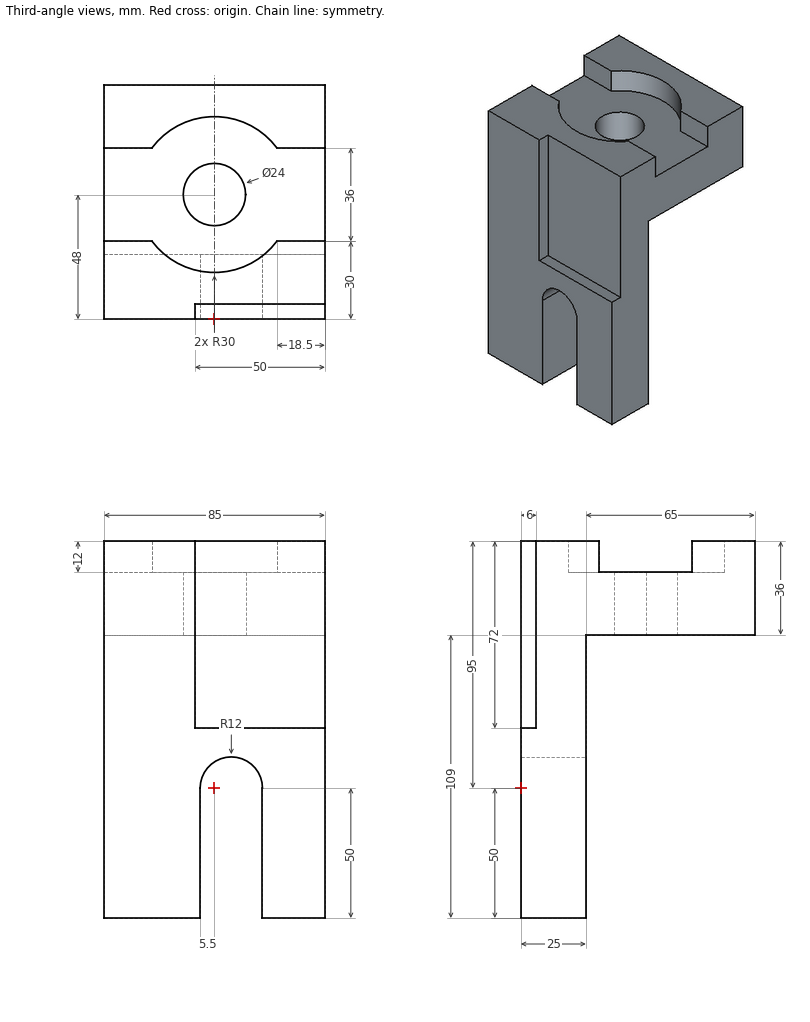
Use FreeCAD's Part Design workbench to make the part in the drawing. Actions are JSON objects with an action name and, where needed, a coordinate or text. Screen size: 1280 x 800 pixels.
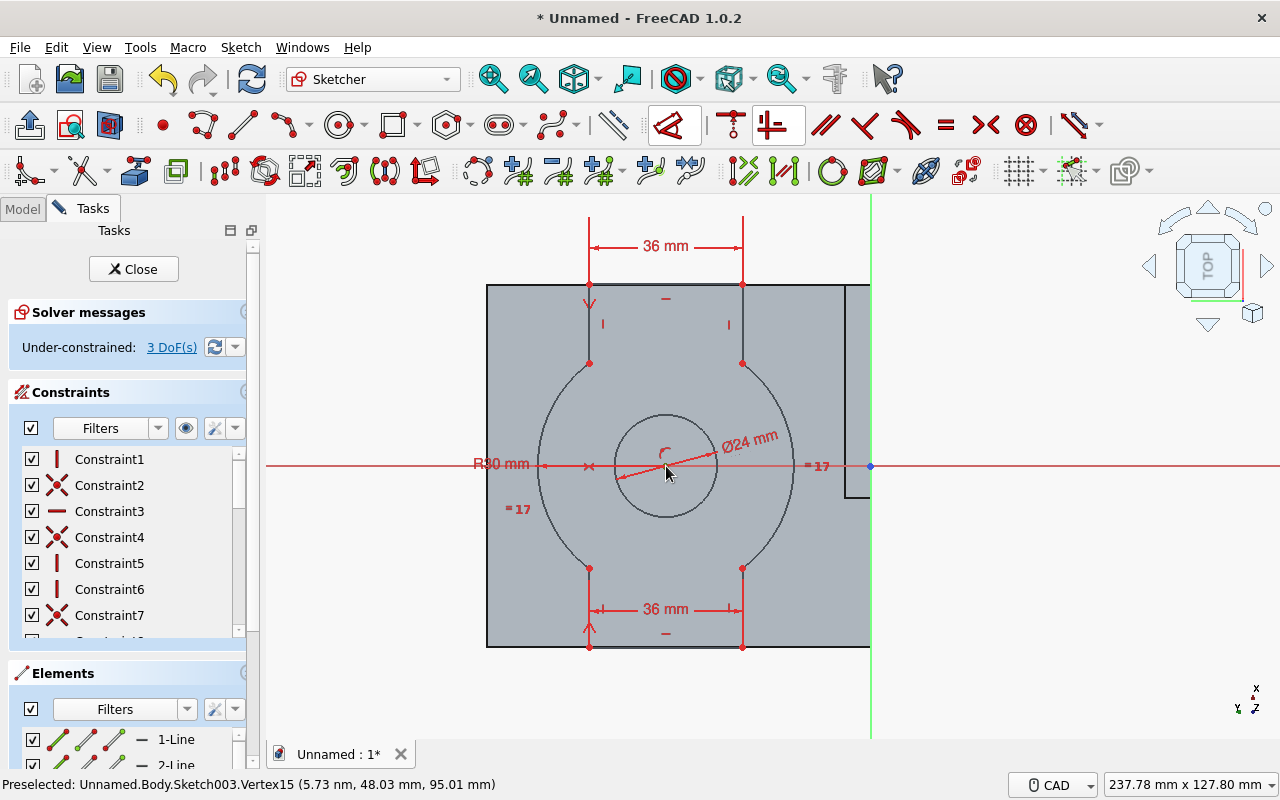
{"action": "left_click", "coordinate": [696, 126]}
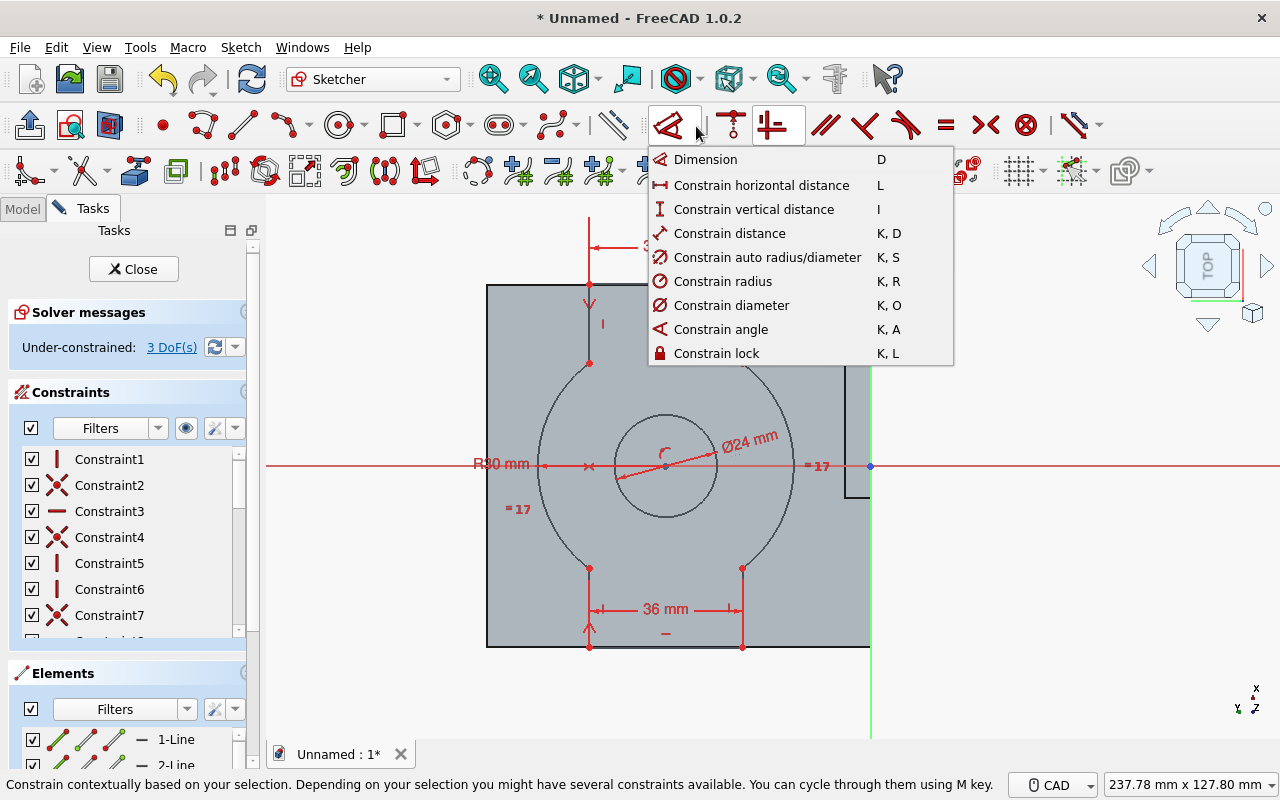
{"action": "left_click", "coordinate": [801, 185]}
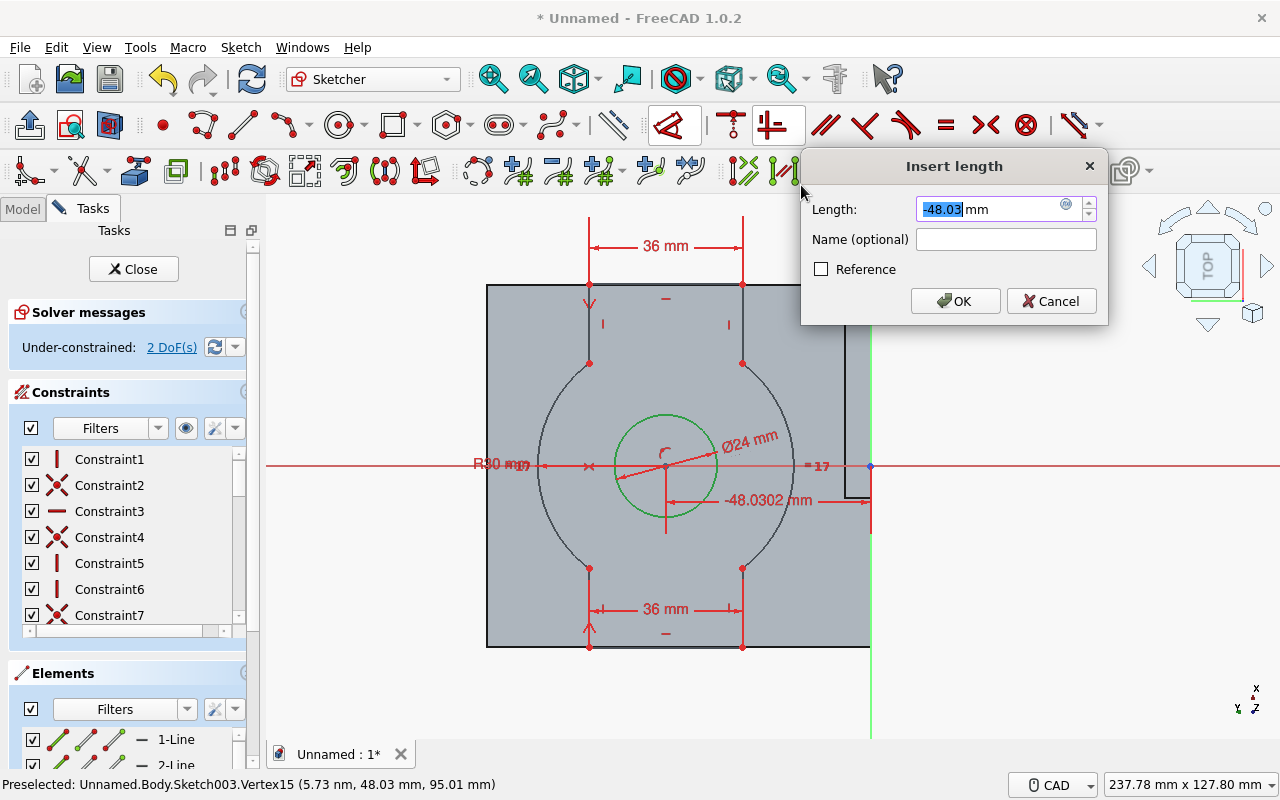
{"action": "type", "text": "-48"}
{"action": "key", "text": "Return"}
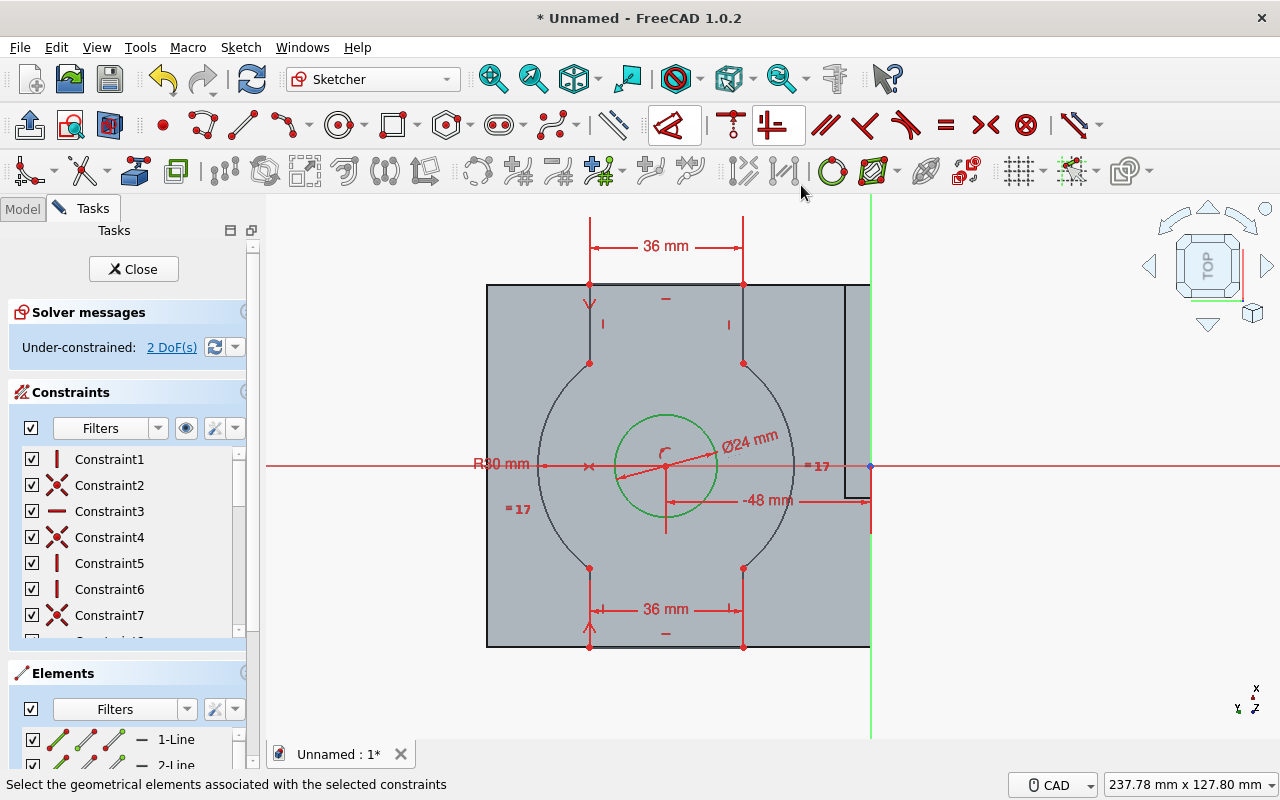
{"action": "left_click", "coordinate": [743, 364]}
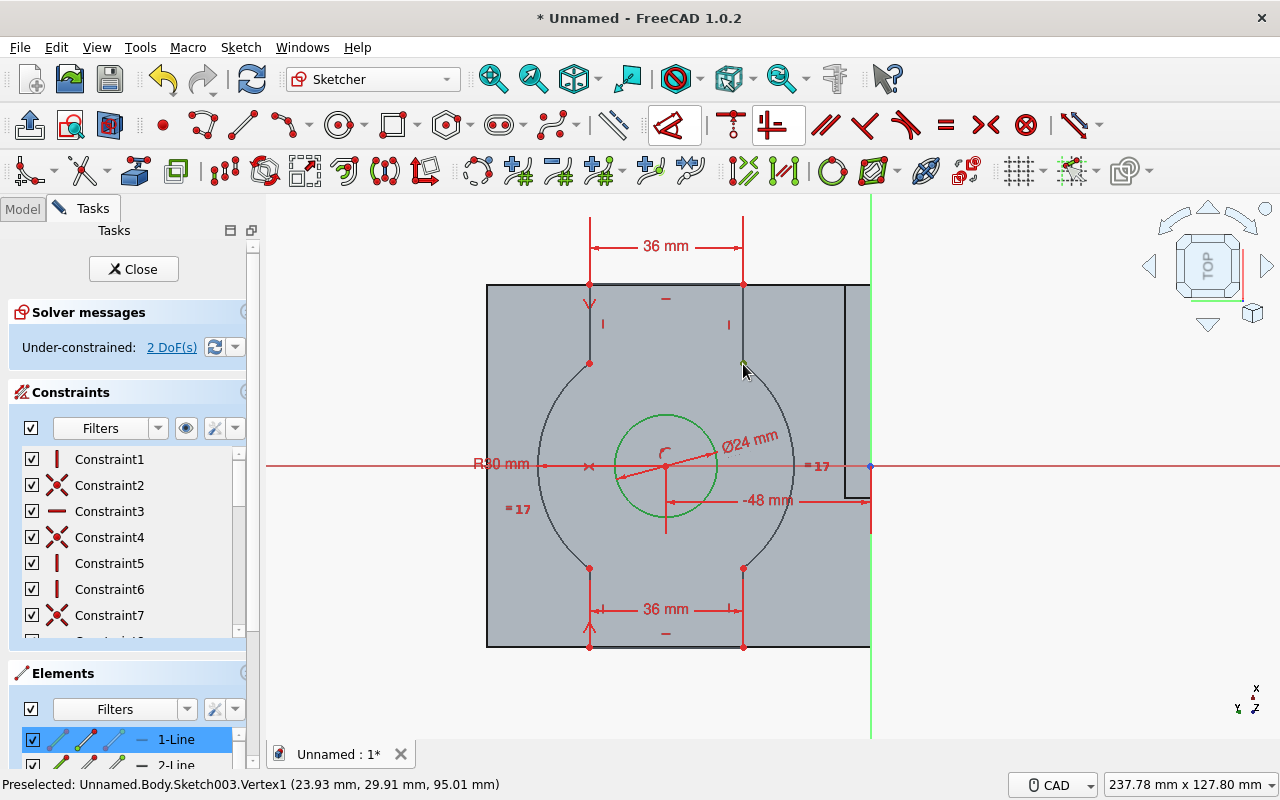
{"action": "left_click", "coordinate": [696, 126]}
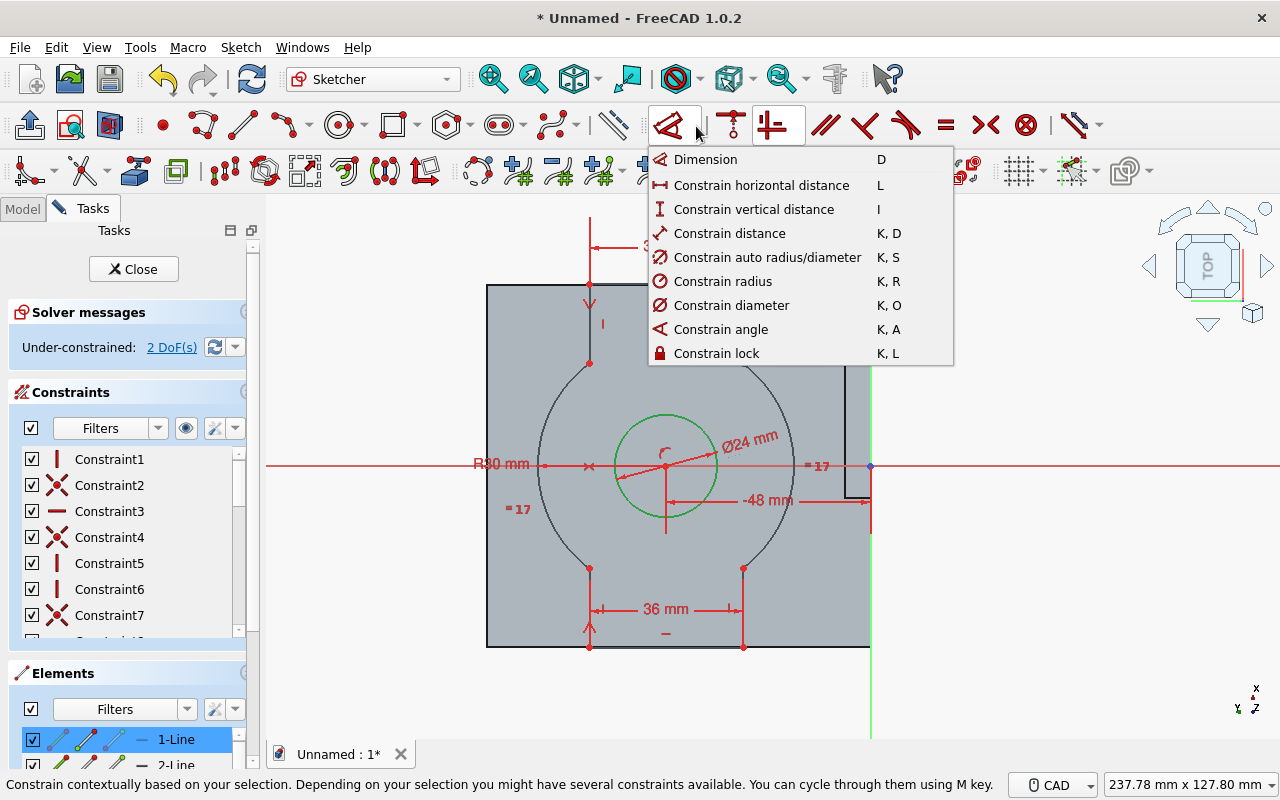
{"action": "left_click", "coordinate": [801, 185]}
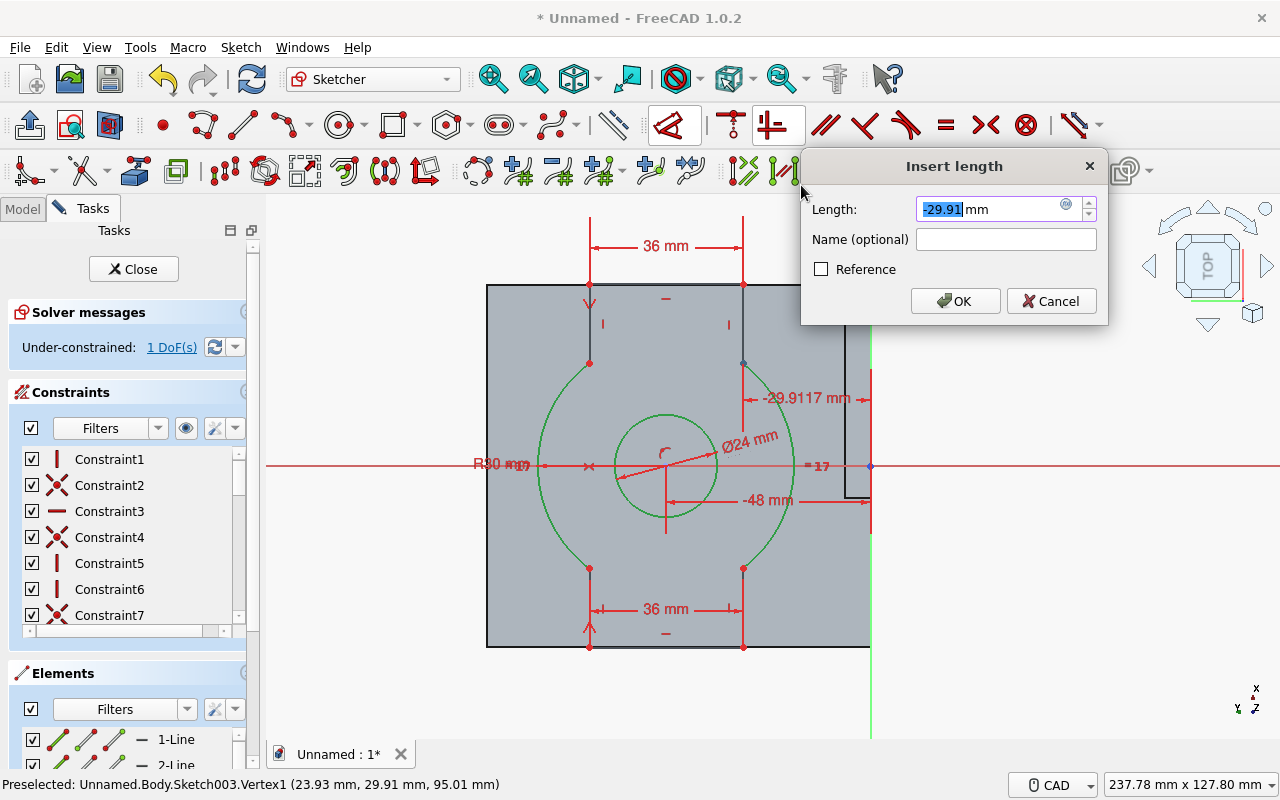
{"action": "type", "text": "-30"}
{"action": "key", "text": "Return"}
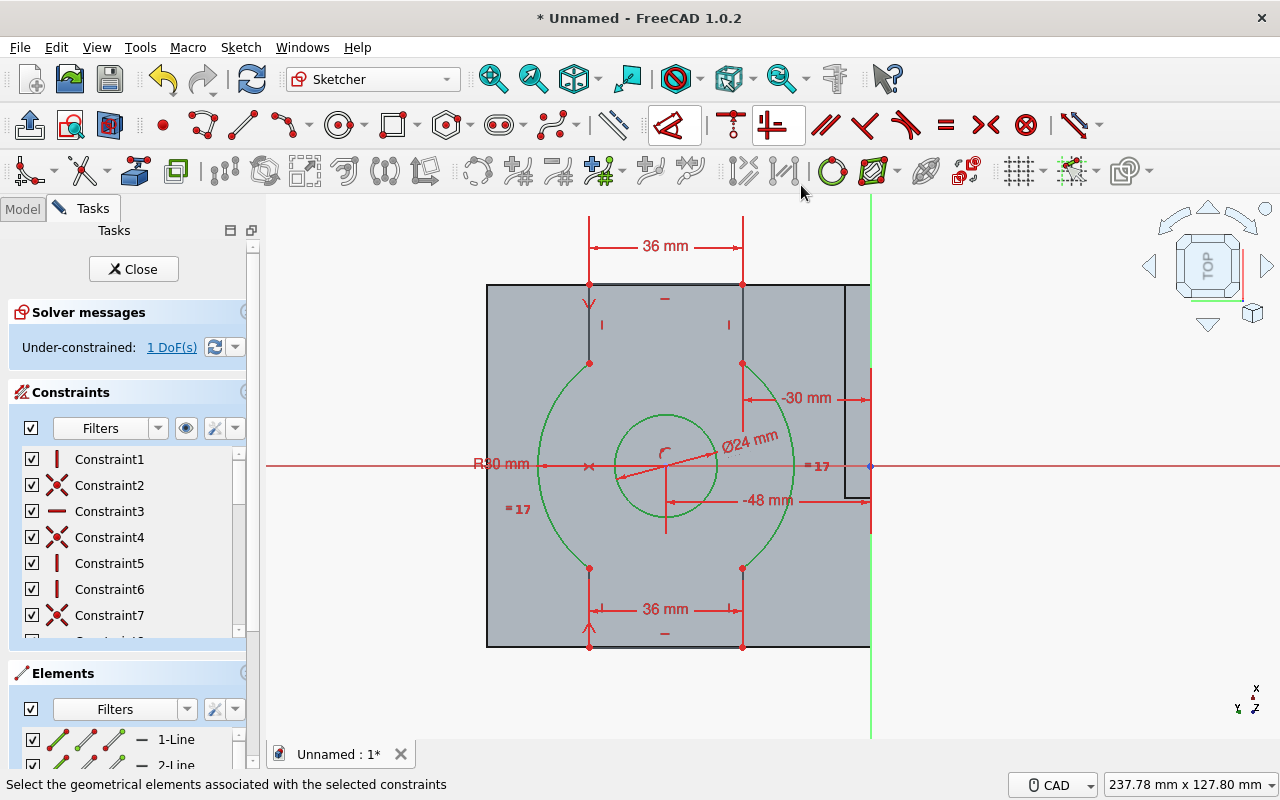
{"action": "left_click", "coordinate": [743, 340]}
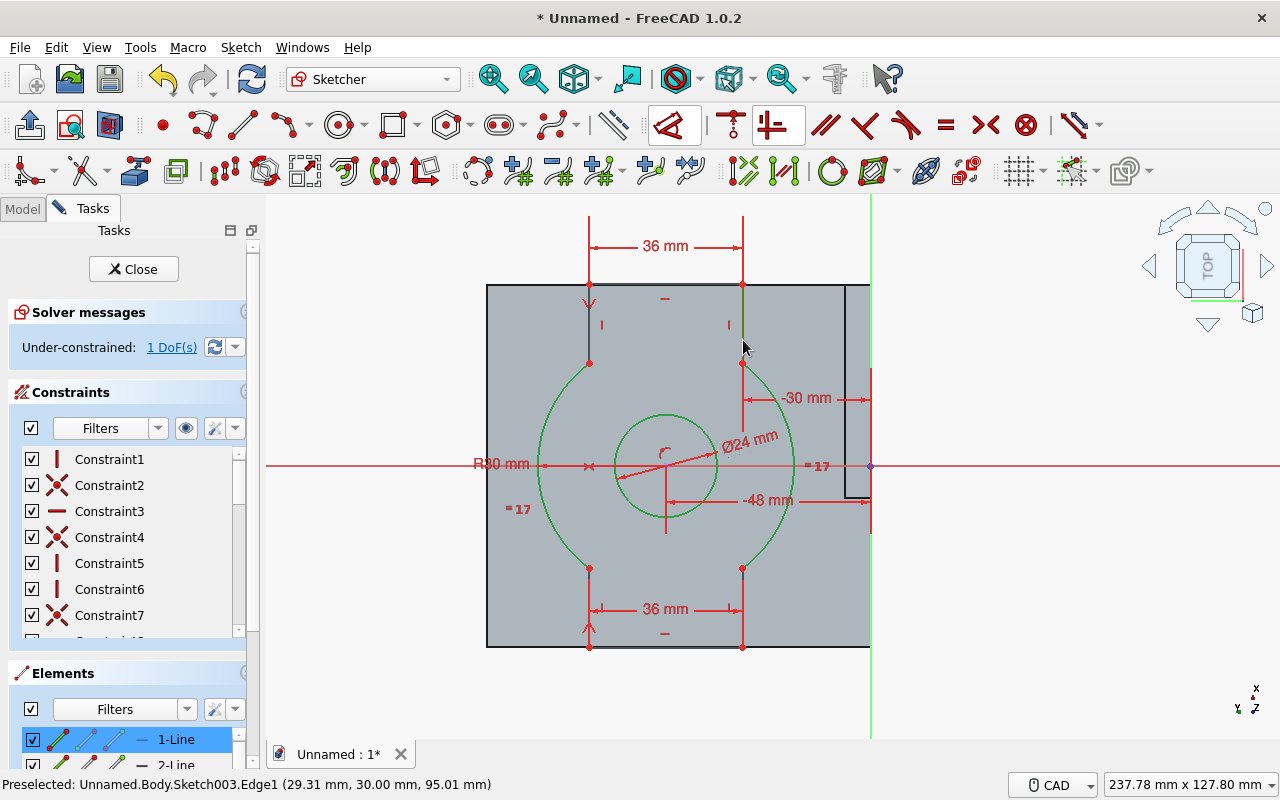
{"action": "left_click", "coordinate": [696, 126]}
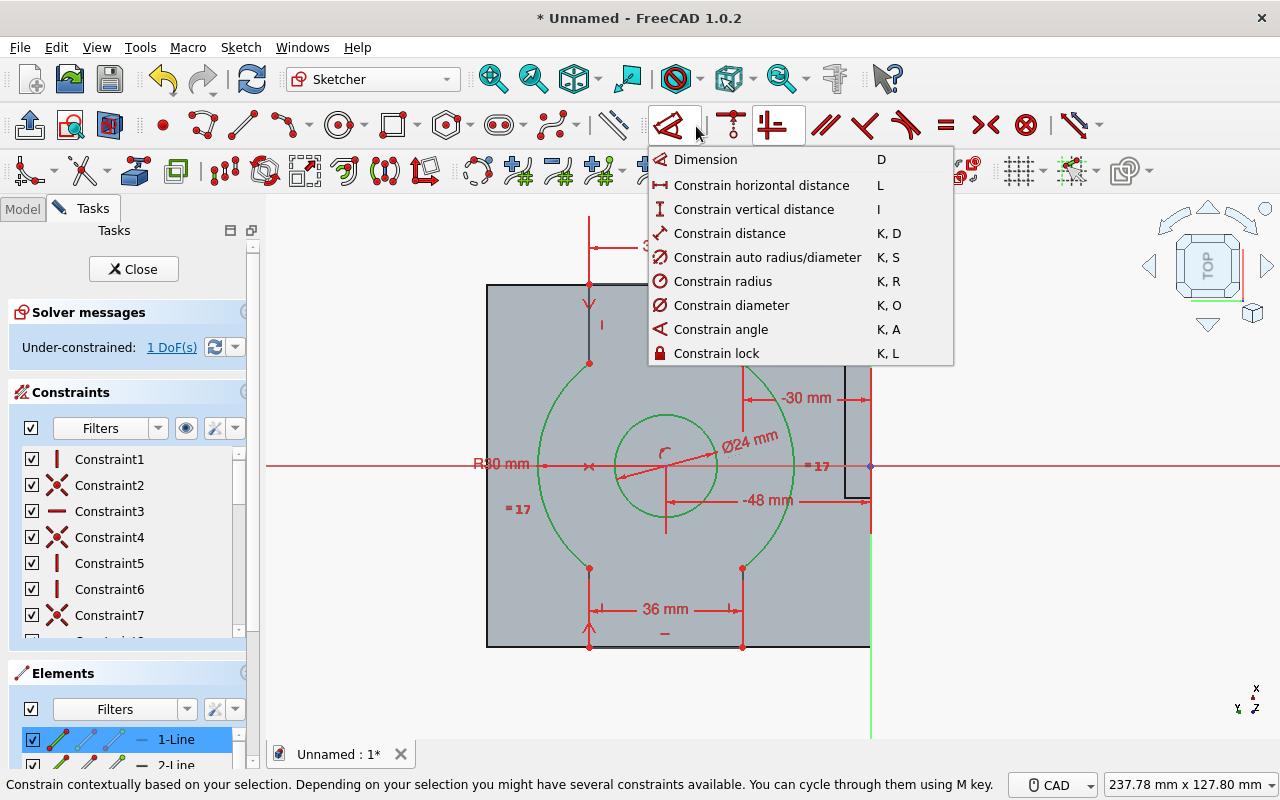
{"action": "left_click", "coordinate": [801, 209]}